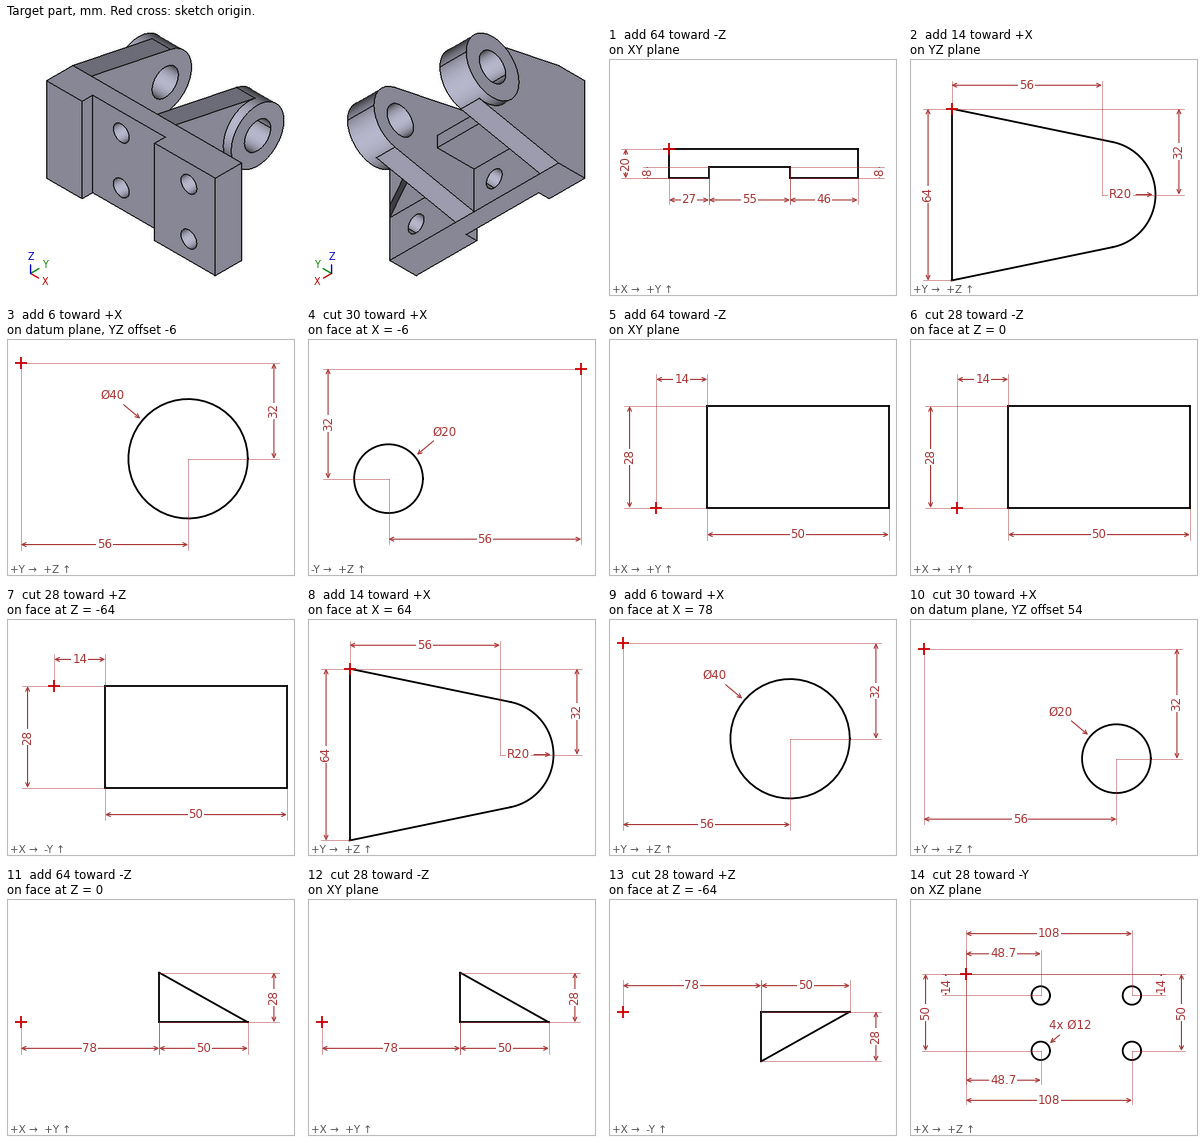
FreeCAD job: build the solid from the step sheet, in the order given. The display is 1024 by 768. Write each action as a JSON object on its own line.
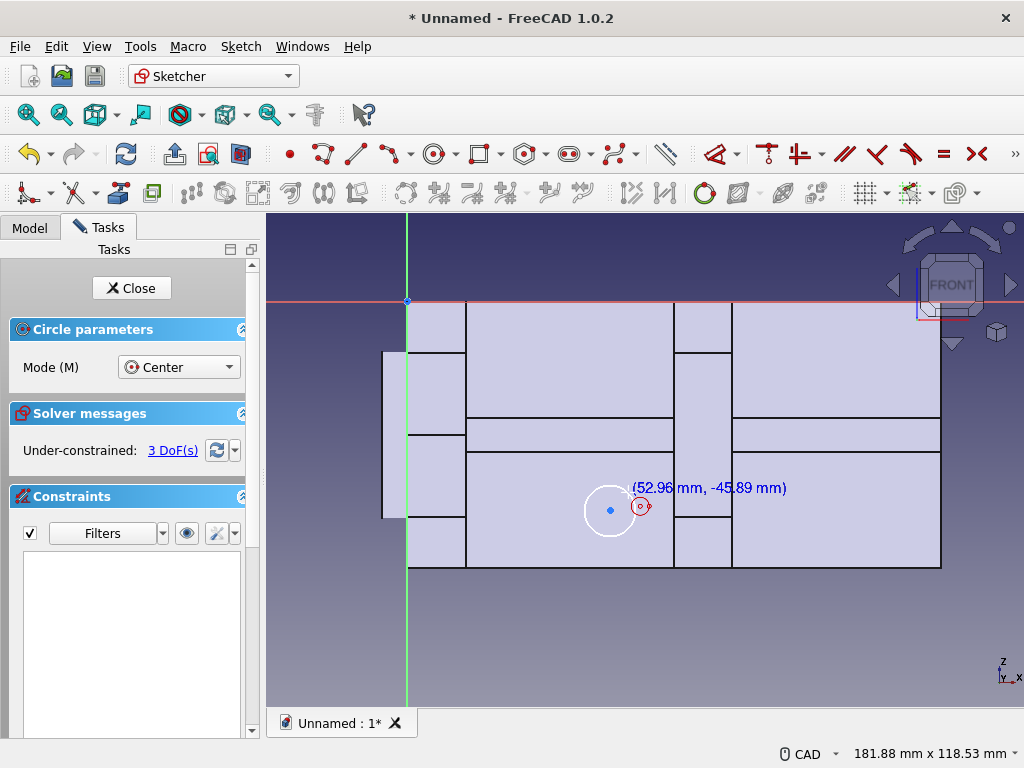
{"action": "left_click", "coordinate": [857, 510]}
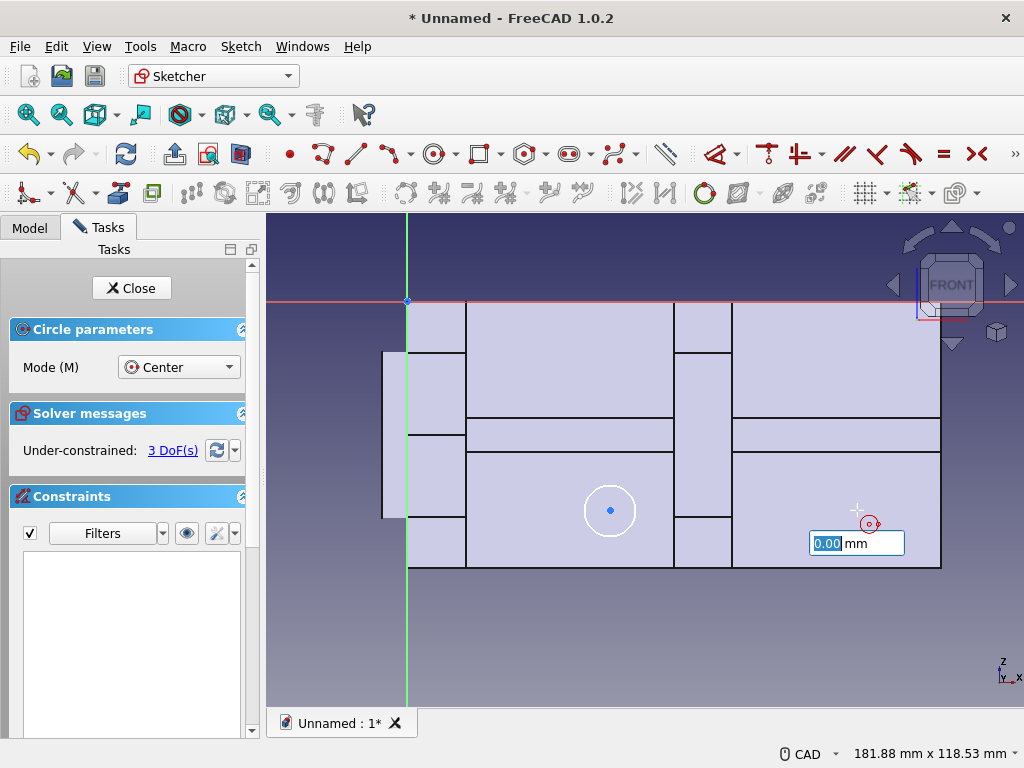
{"action": "scroll", "coordinate": [294, 648], "scroll_direction": "down", "scroll_amount": 1}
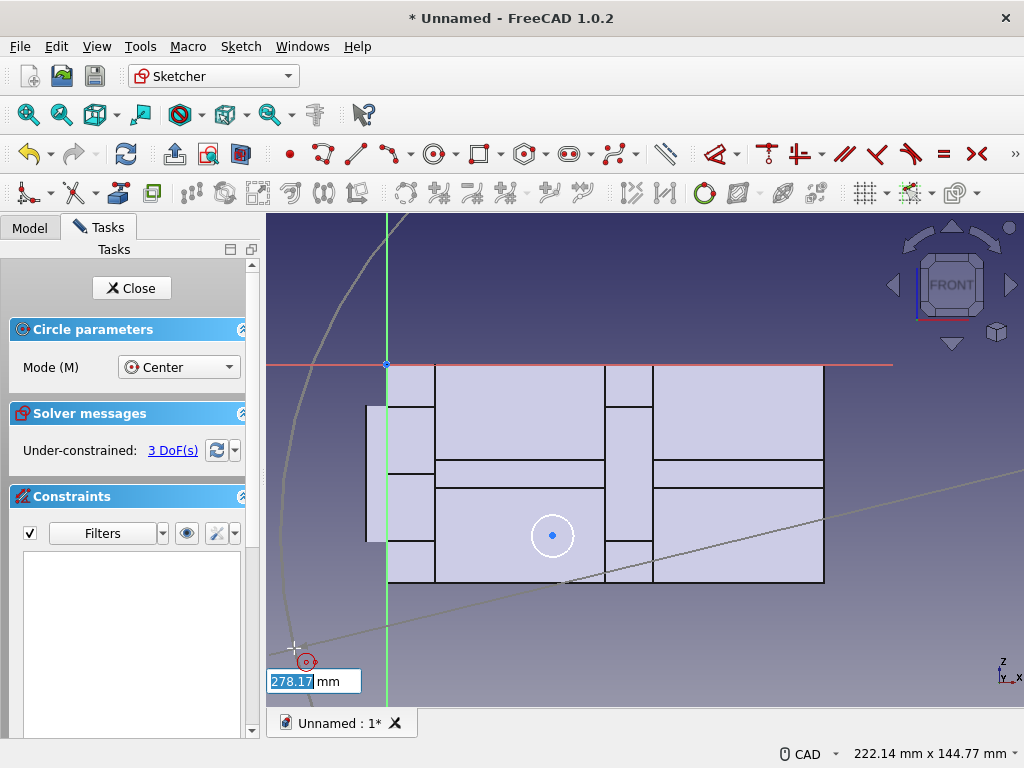
{"action": "left_click", "coordinate": [770, 521]}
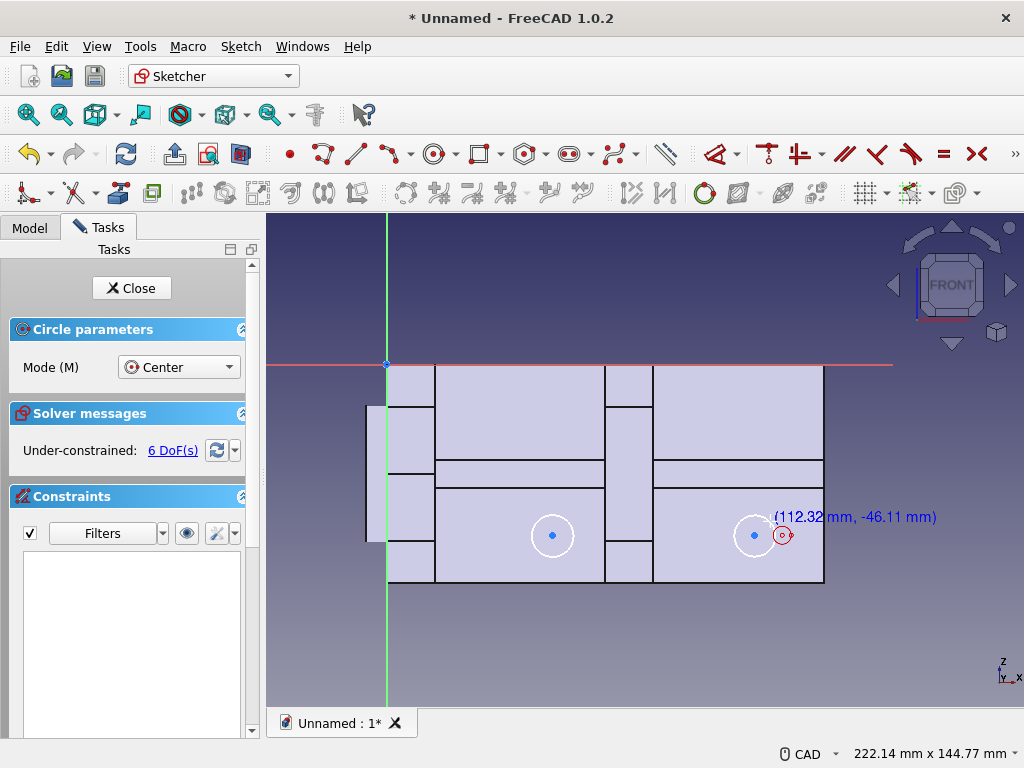
{"action": "left_click", "coordinate": [755, 412]}
{"action": "left_click", "coordinate": [770, 398]}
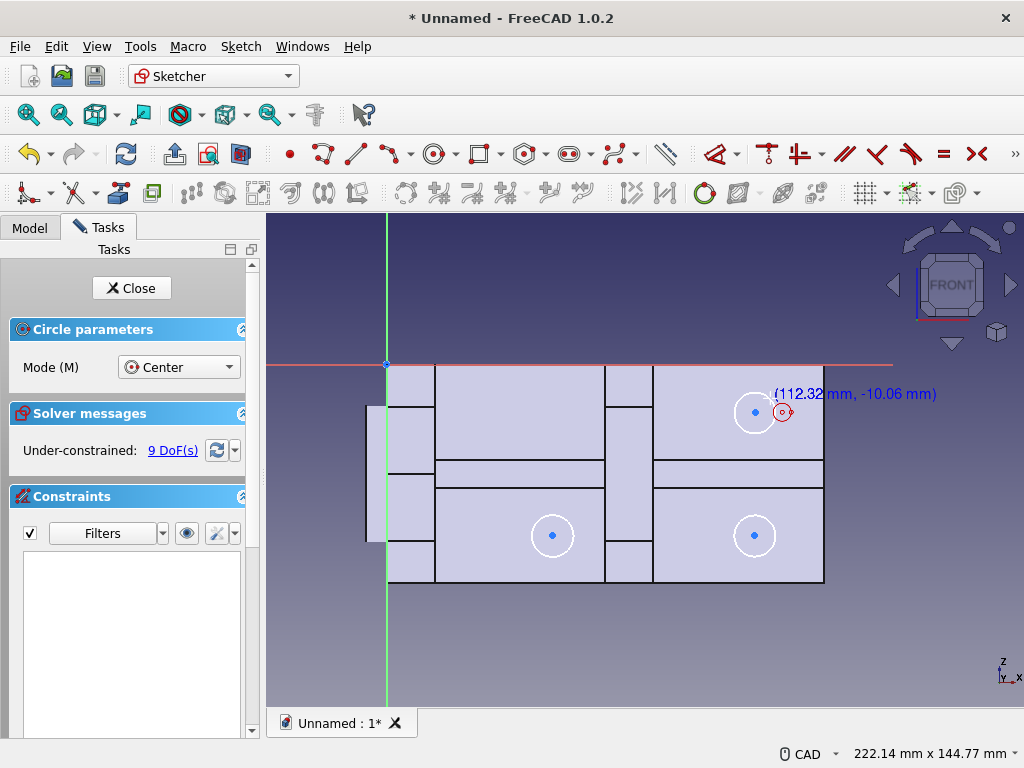
{"action": "left_click", "coordinate": [553, 412]}
{"action": "left_click", "coordinate": [567, 398]}
{"action": "key", "text": "Escape"}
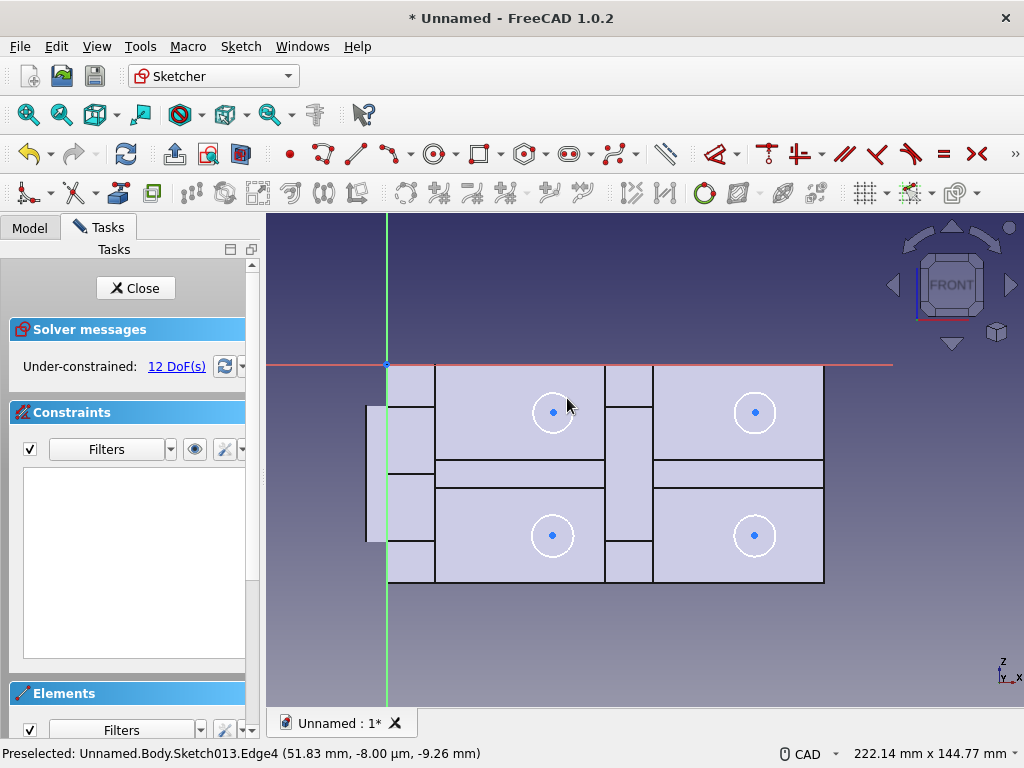
{"action": "left_click", "coordinate": [567, 521]}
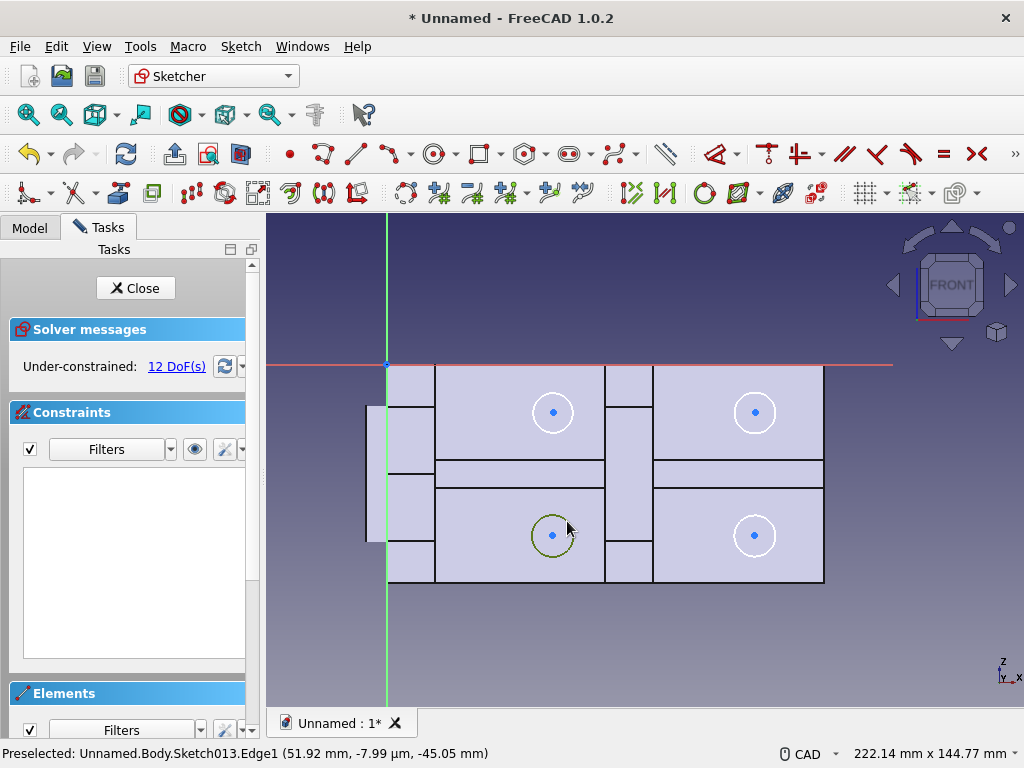
{"action": "left_click", "coordinate": [769, 521]}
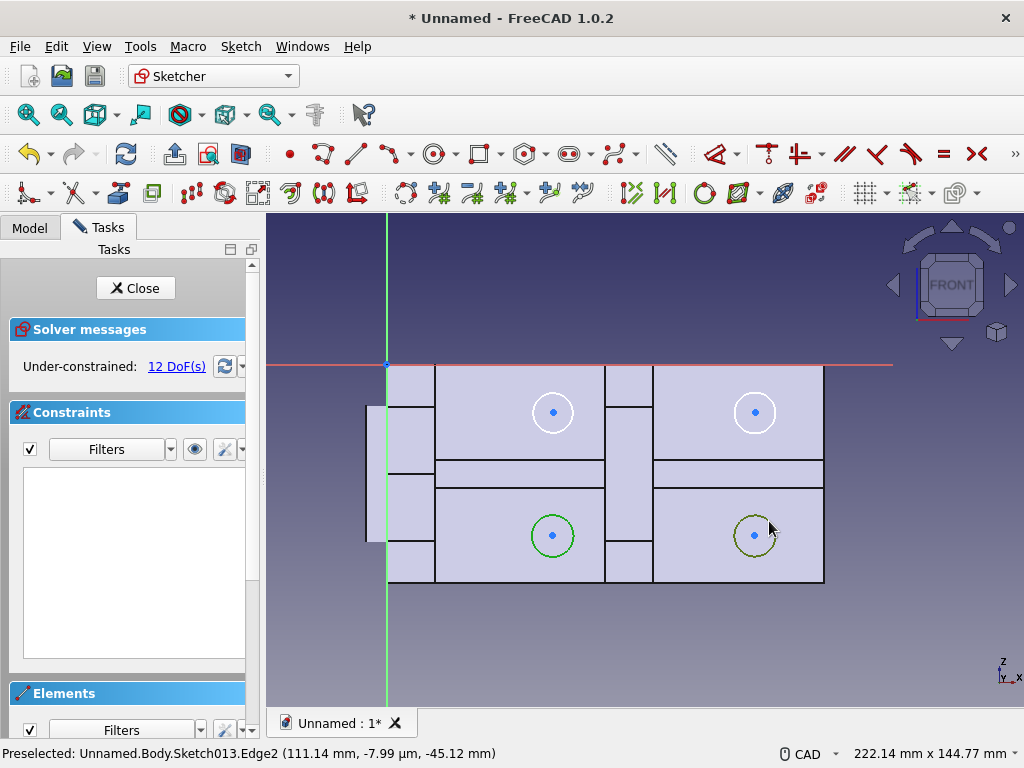
{"action": "left_click", "coordinate": [769, 398]}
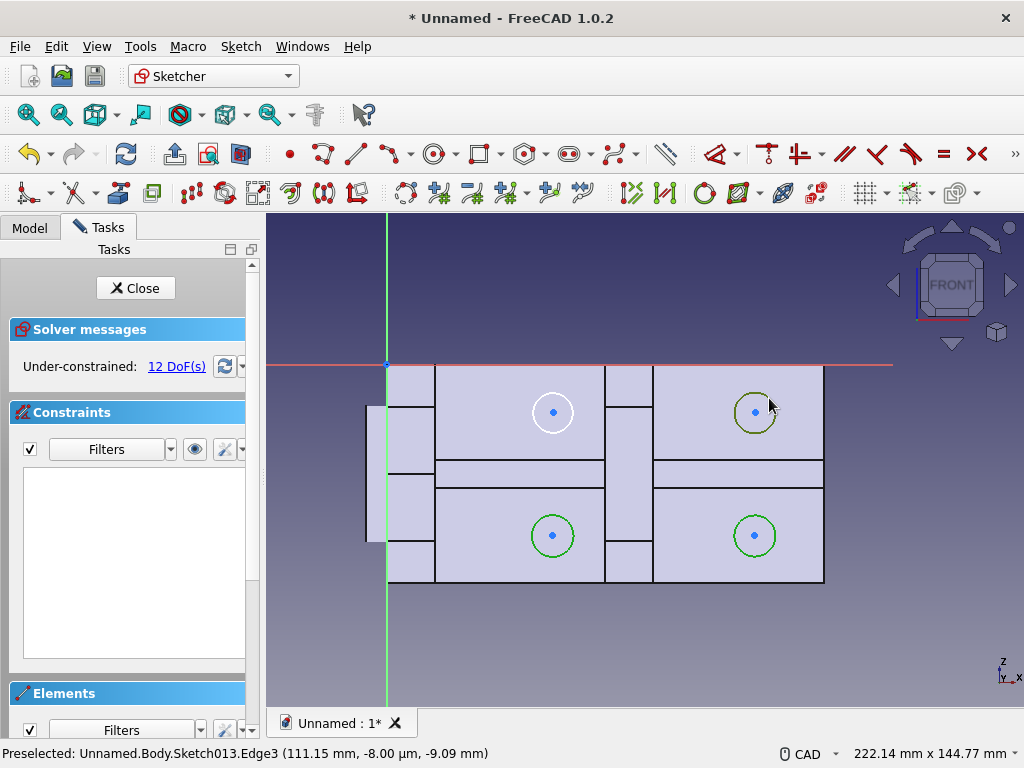
{"action": "left_click", "coordinate": [567, 399]}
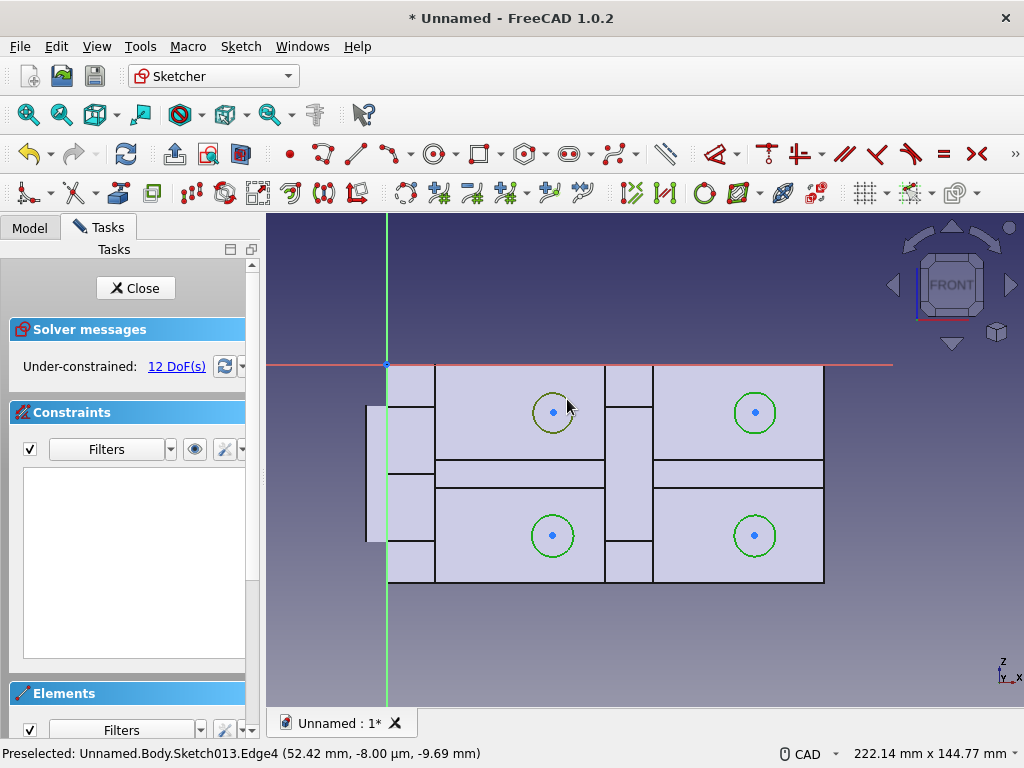
{"action": "left_click", "coordinate": [944, 154]}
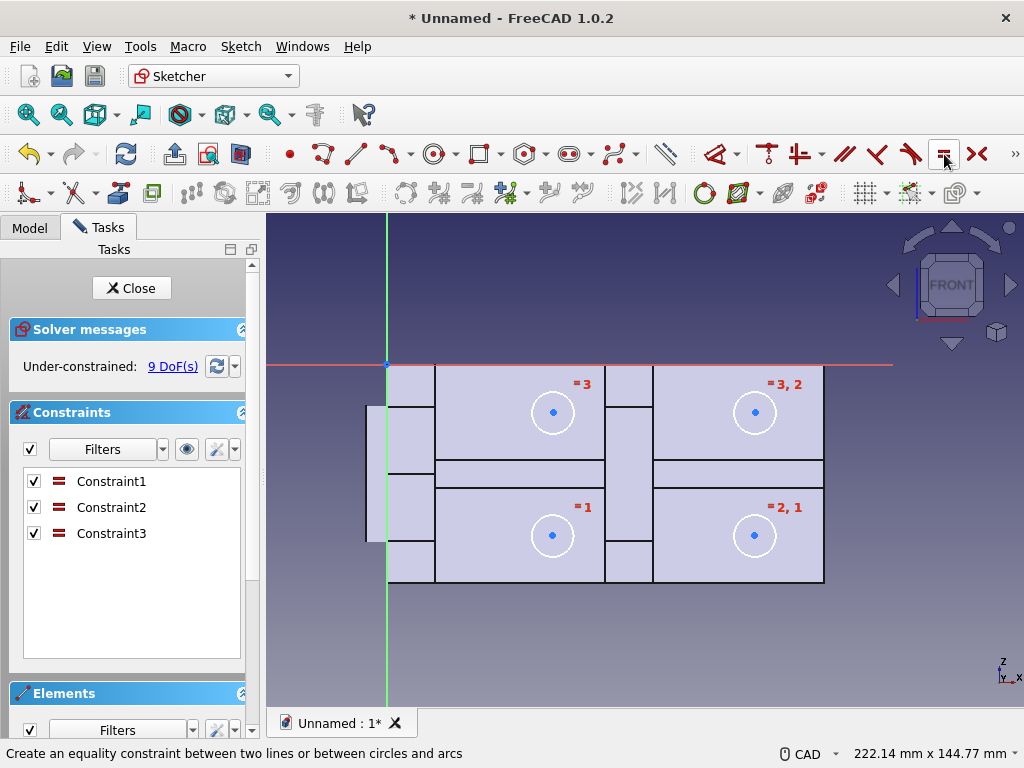
{"action": "left_click", "coordinate": [714, 154]}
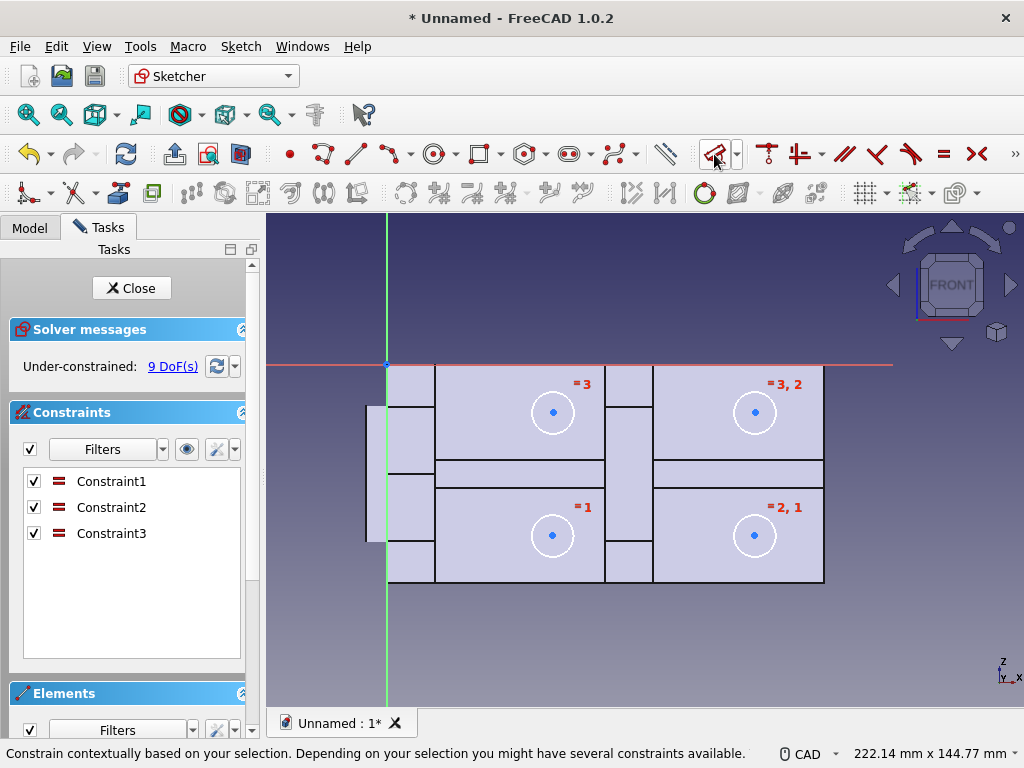
{"action": "left_click", "coordinate": [567, 521]}
{"action": "left_click", "coordinate": [589, 498]}